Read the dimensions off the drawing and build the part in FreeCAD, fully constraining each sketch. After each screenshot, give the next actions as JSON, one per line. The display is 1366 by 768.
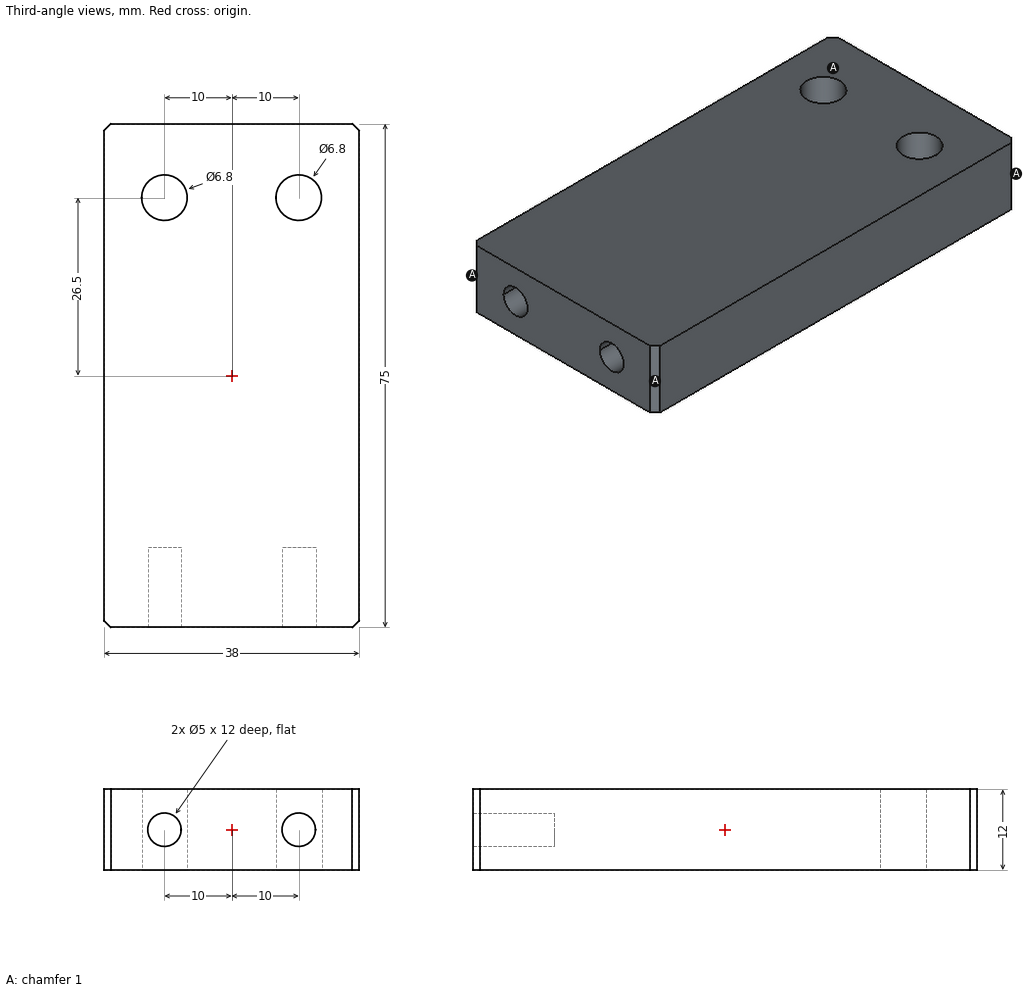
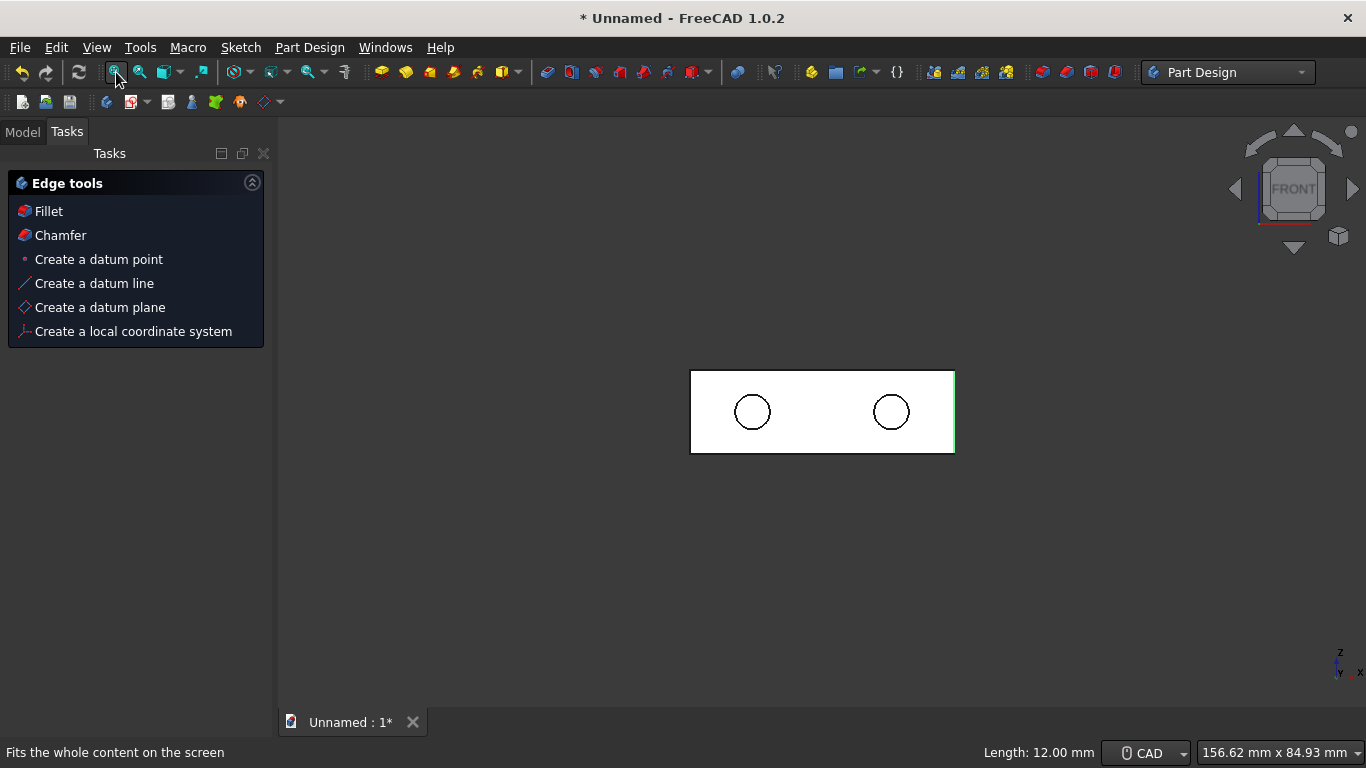
{"action": "left_click", "coordinate": [690, 411], "text": "ctrl"}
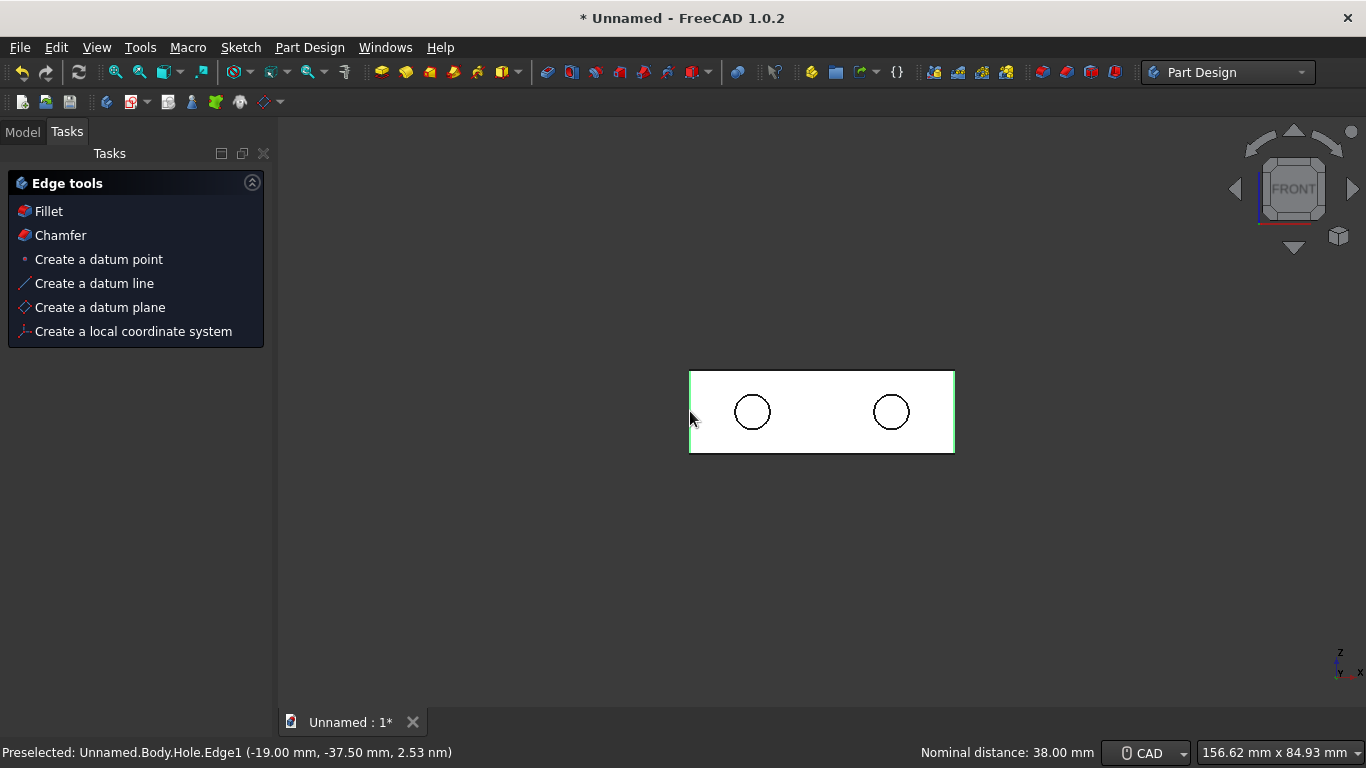
{"action": "key", "text": "3"}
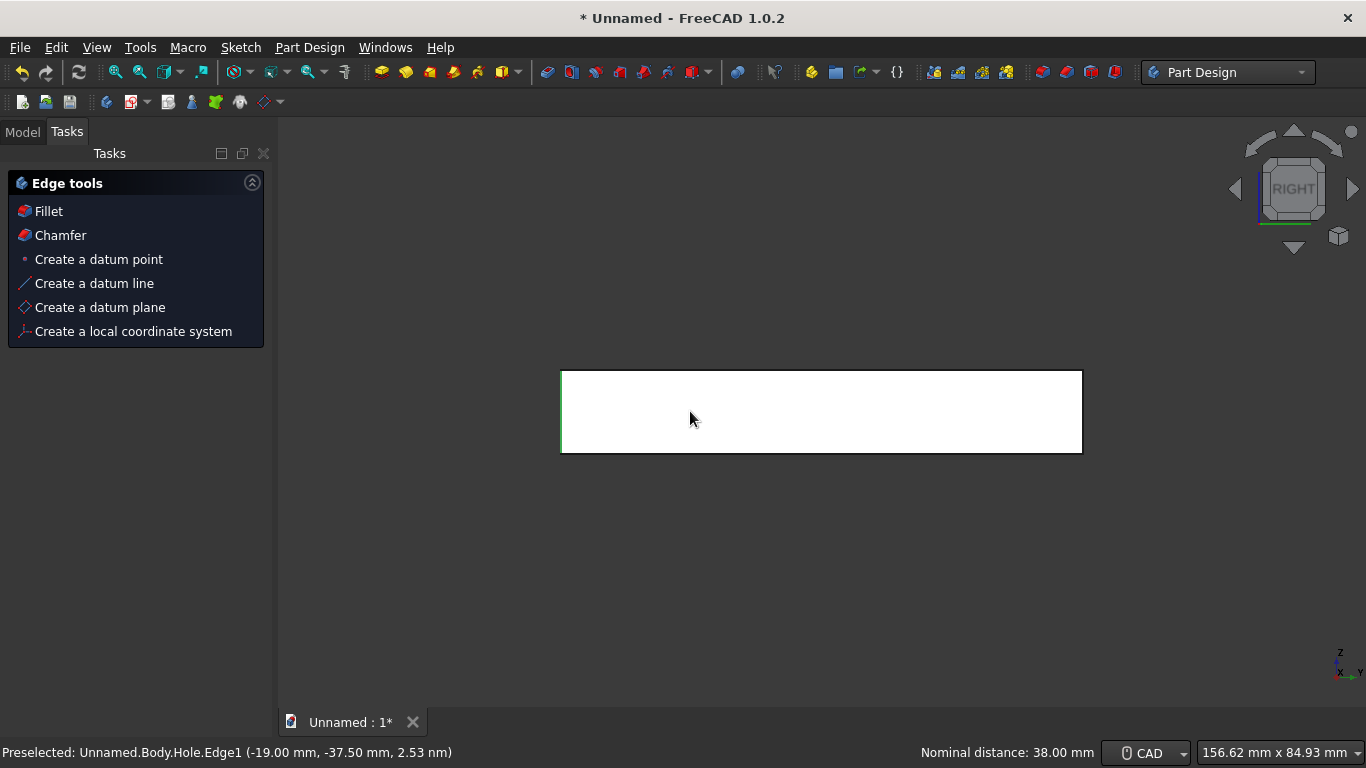
{"action": "left_click", "coordinate": [1083, 411], "text": "ctrl"}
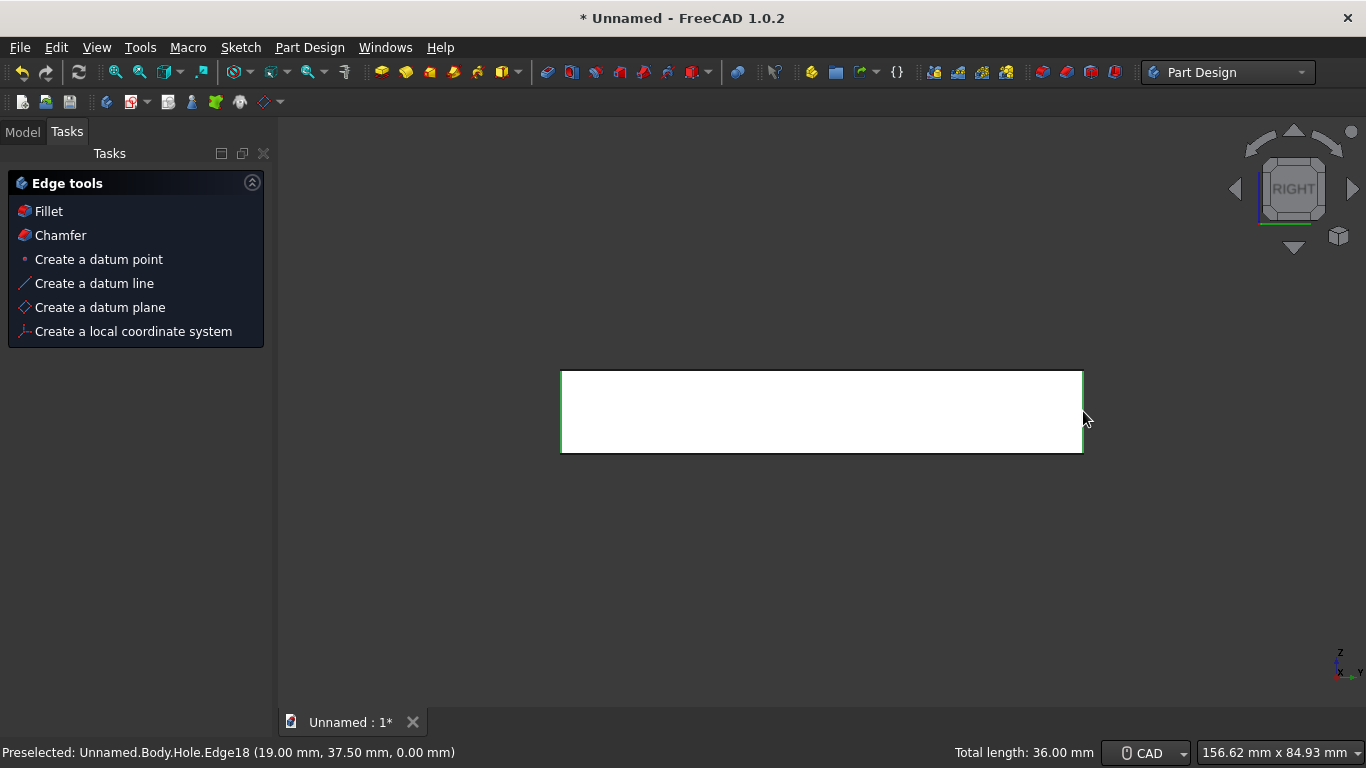
{"action": "key", "text": "5"}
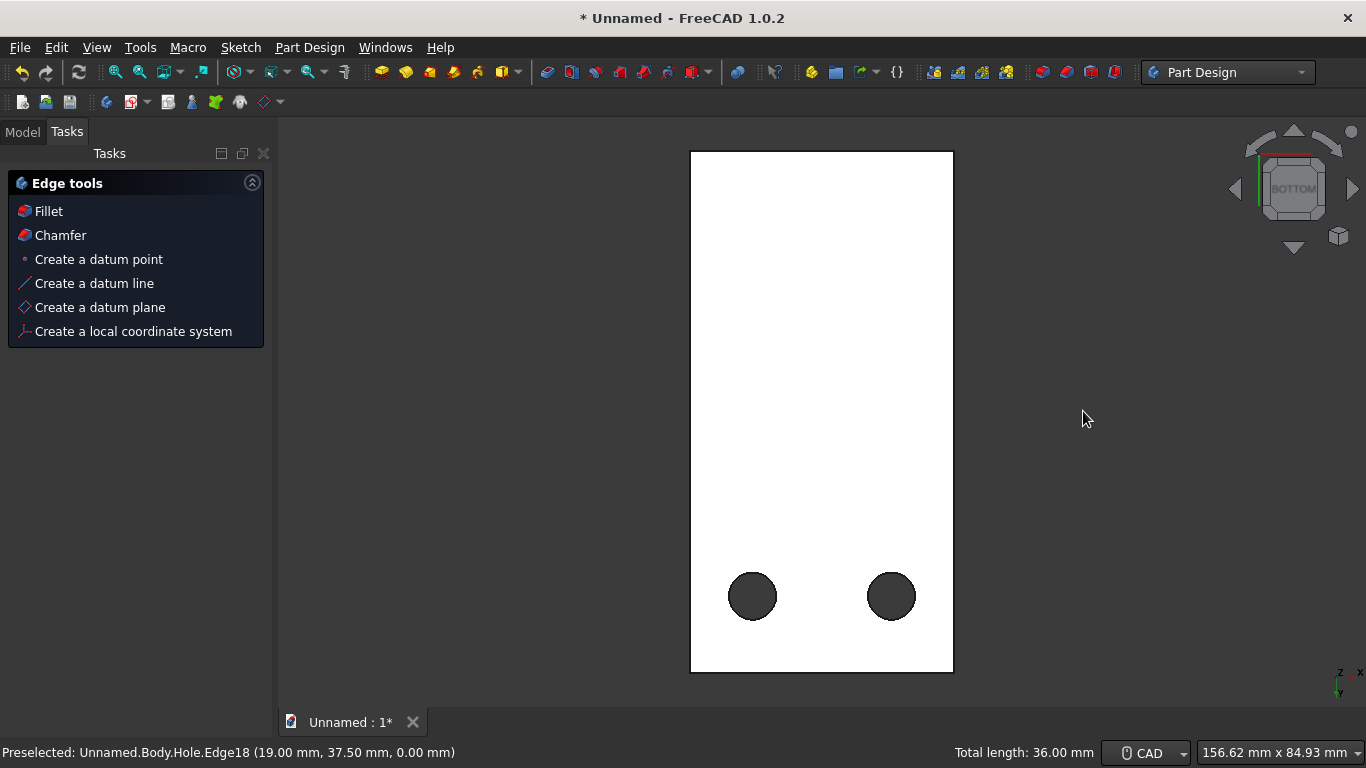
{"action": "key", "text": "4"}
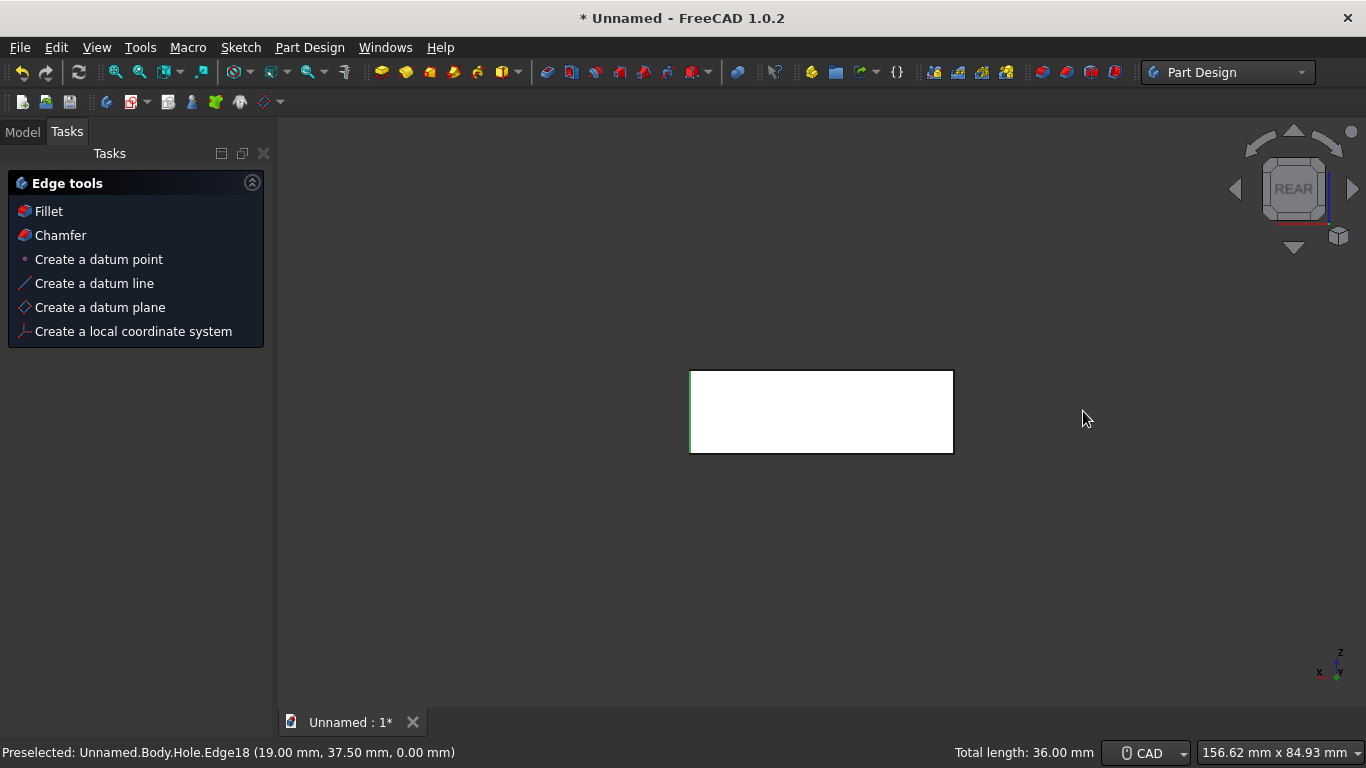
{"action": "key", "text": "v f"}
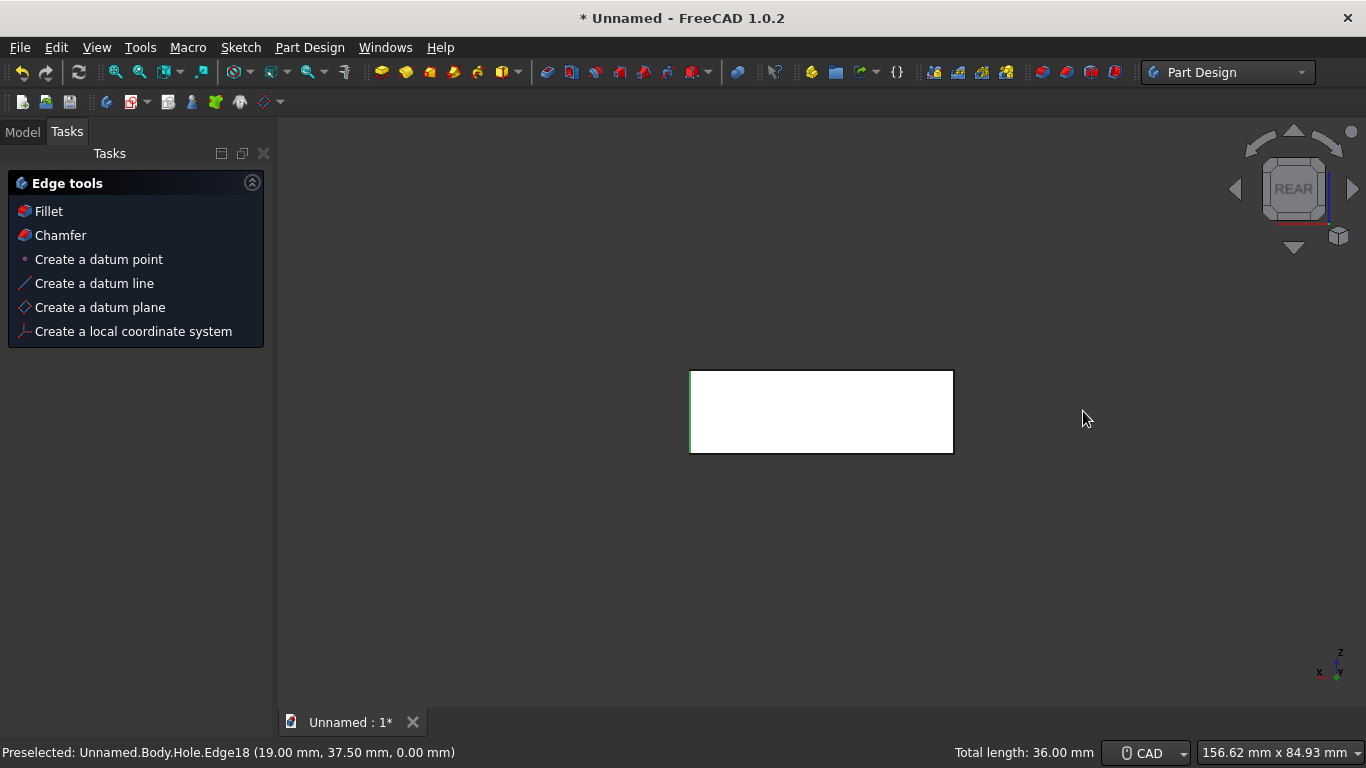
{"action": "left_click", "coordinate": [954, 411], "text": "ctrl"}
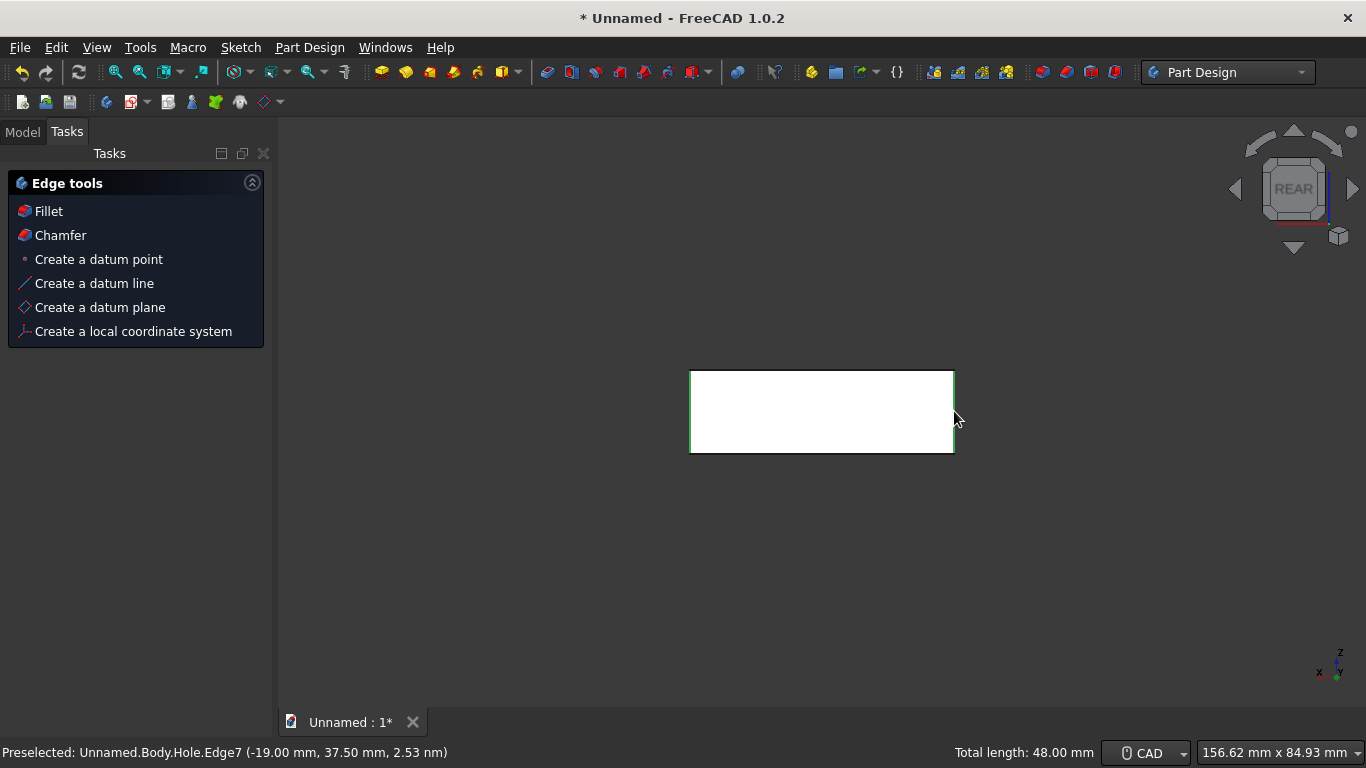
{"action": "left_click", "coordinate": [1068, 72]}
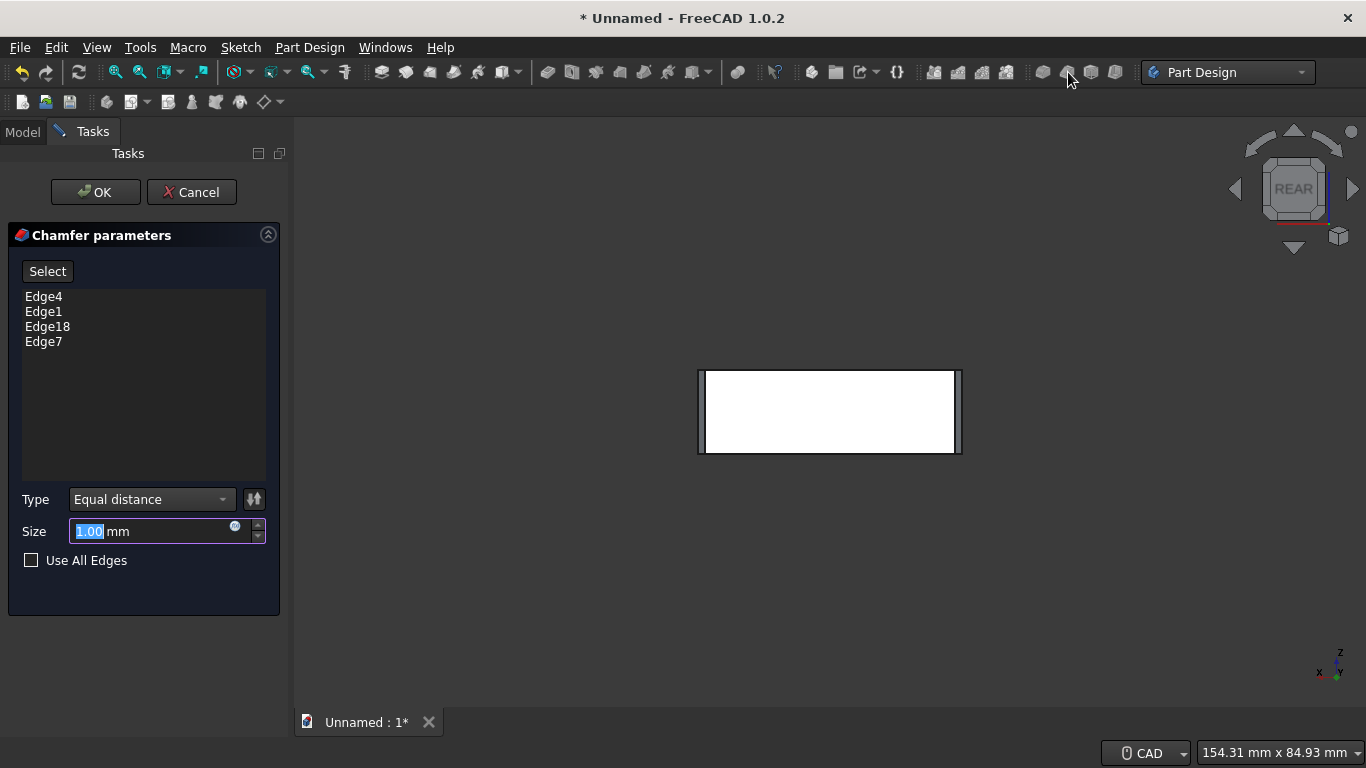
{"action": "type", "text": "1"}
{"action": "key", "text": "Tab"}